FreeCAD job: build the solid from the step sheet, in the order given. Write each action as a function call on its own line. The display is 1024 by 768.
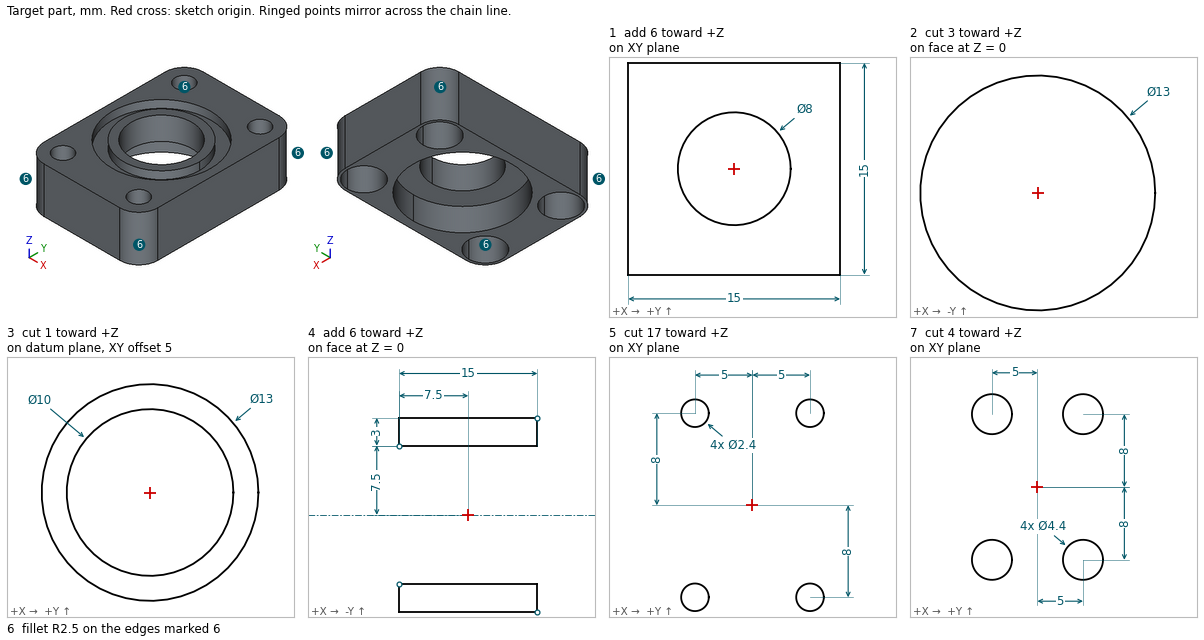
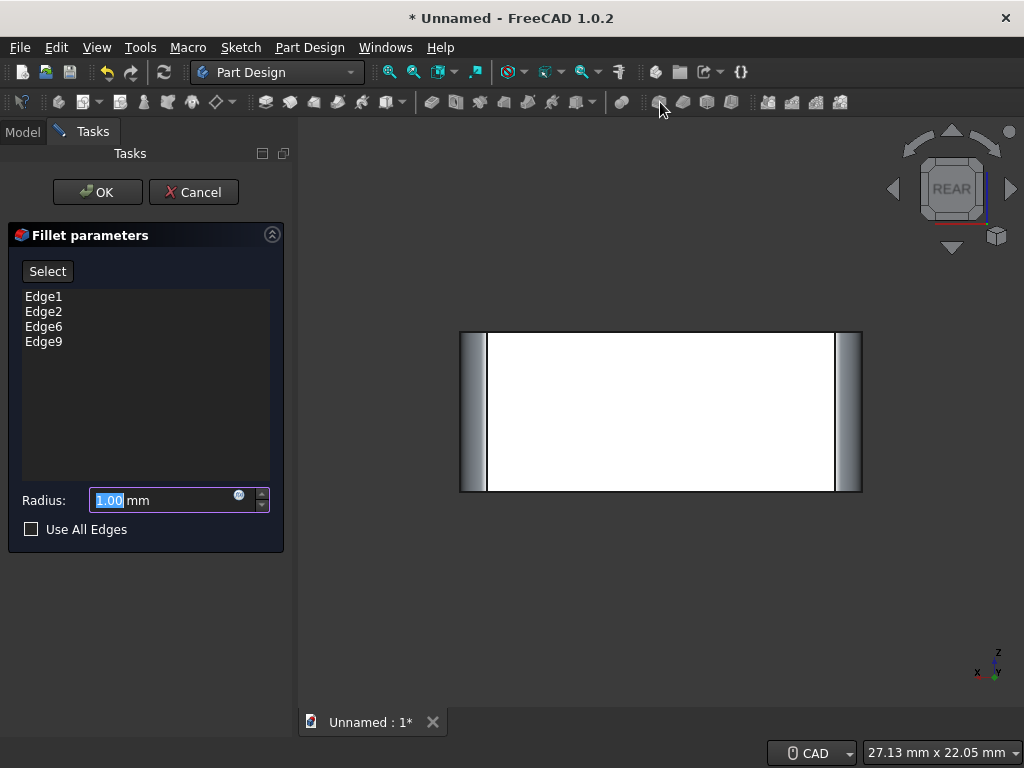
text(2.5)
key(Tab)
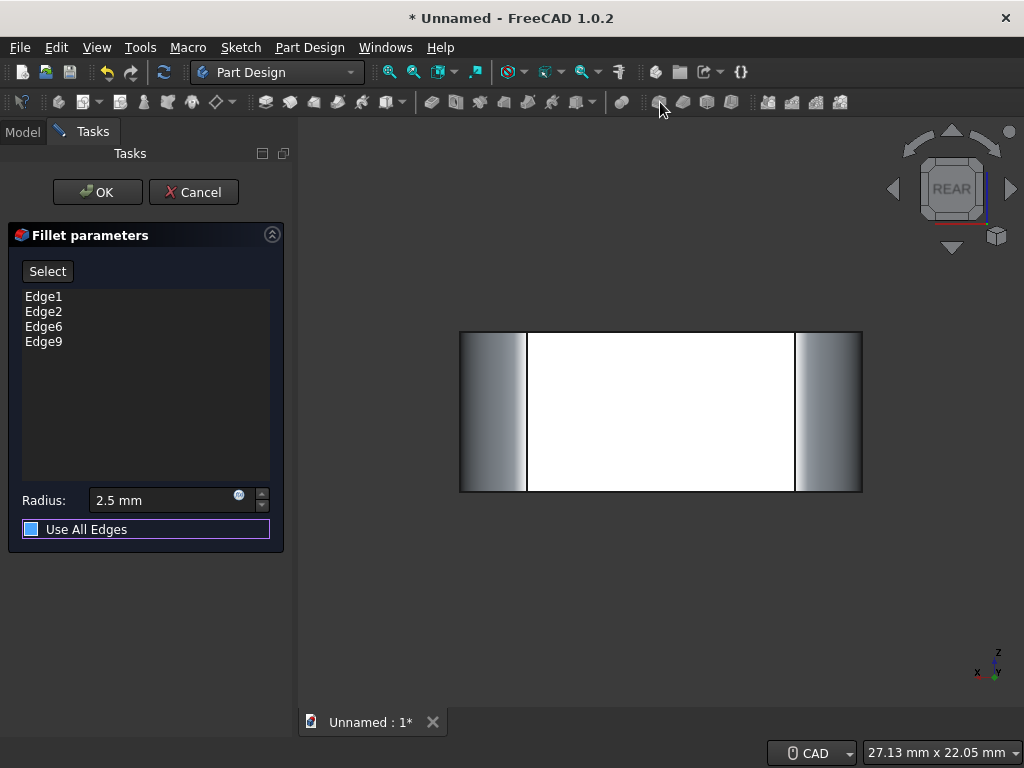
click(98, 192)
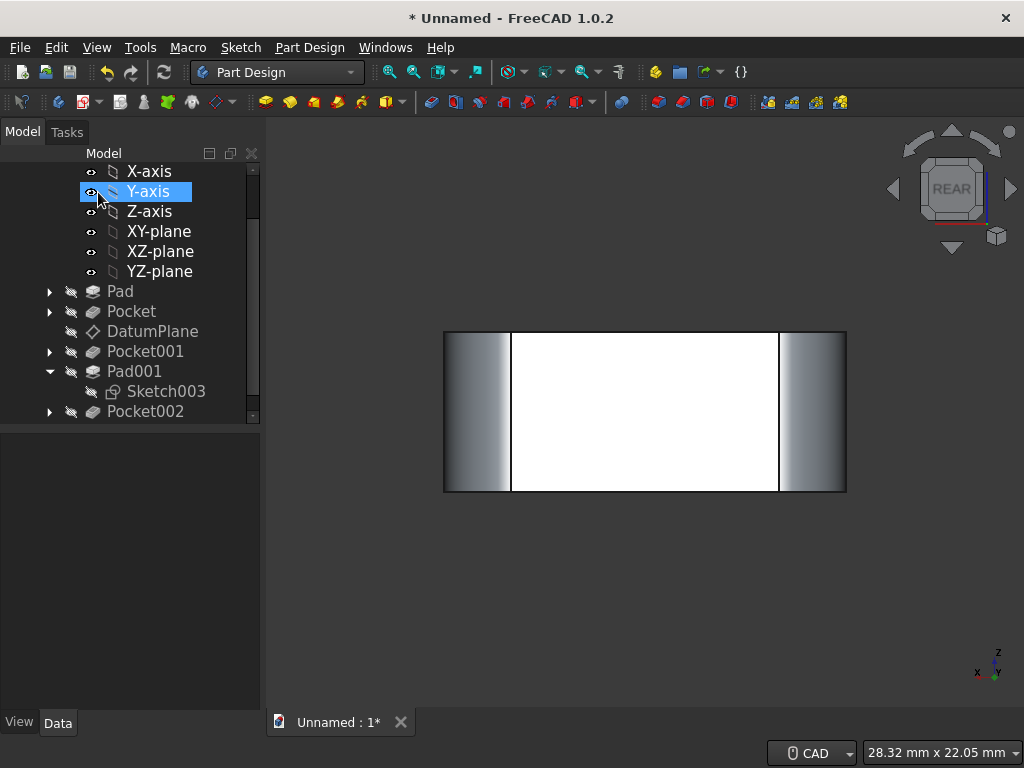
click(84, 102)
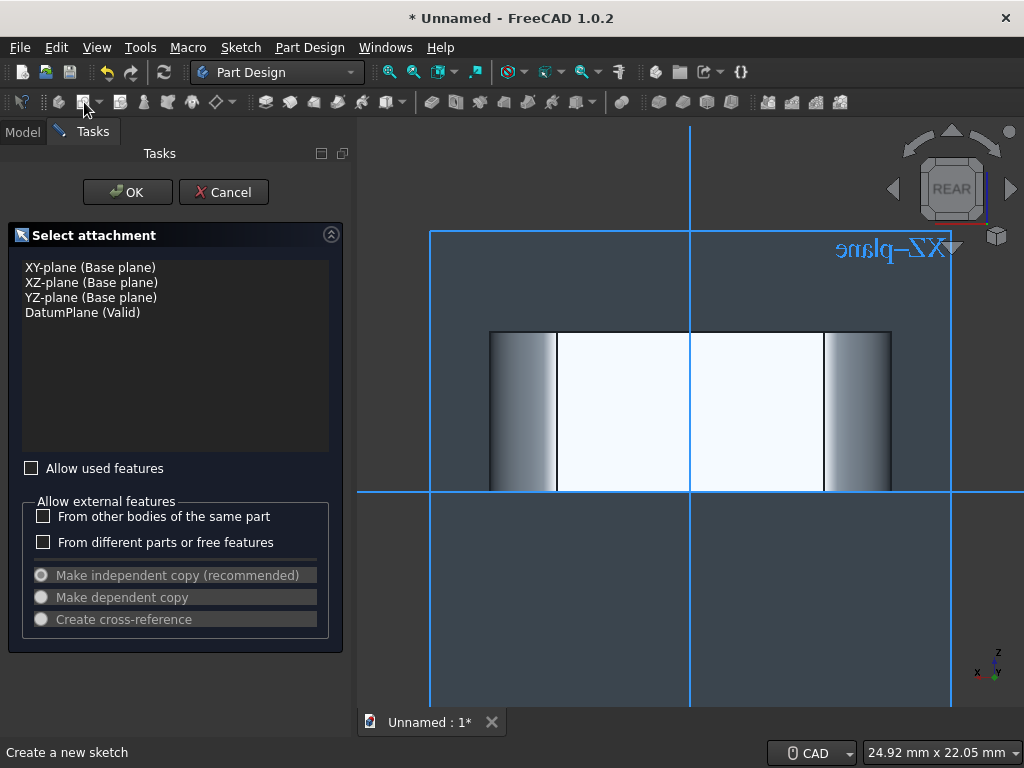
click(82, 268)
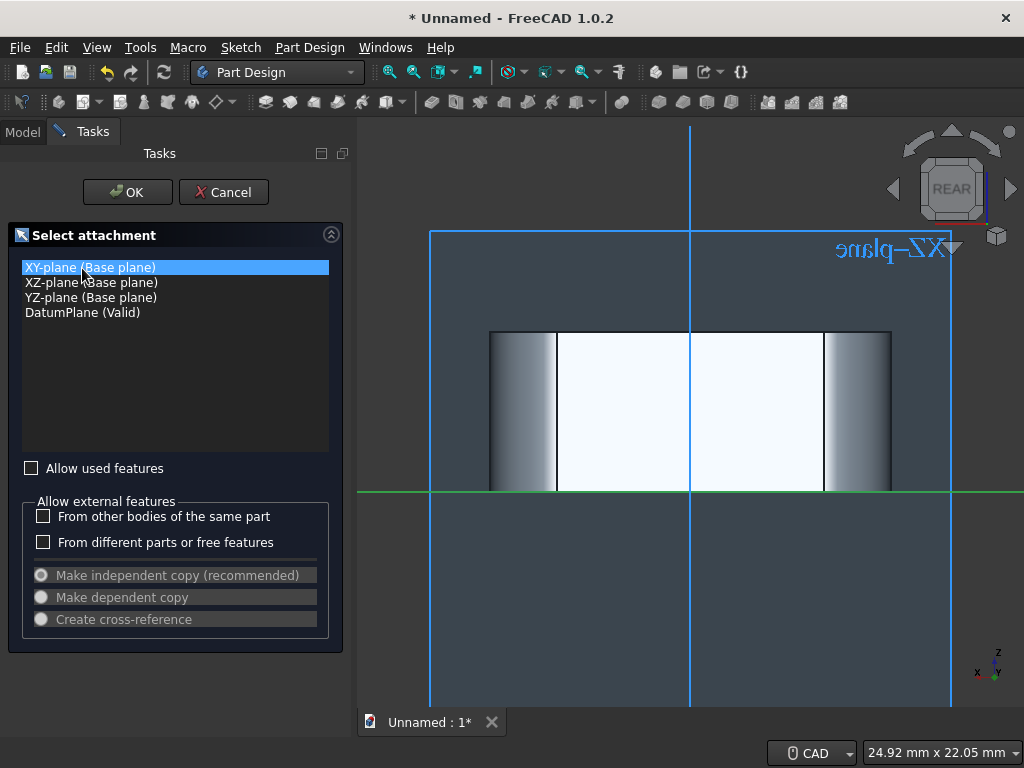
click(128, 192)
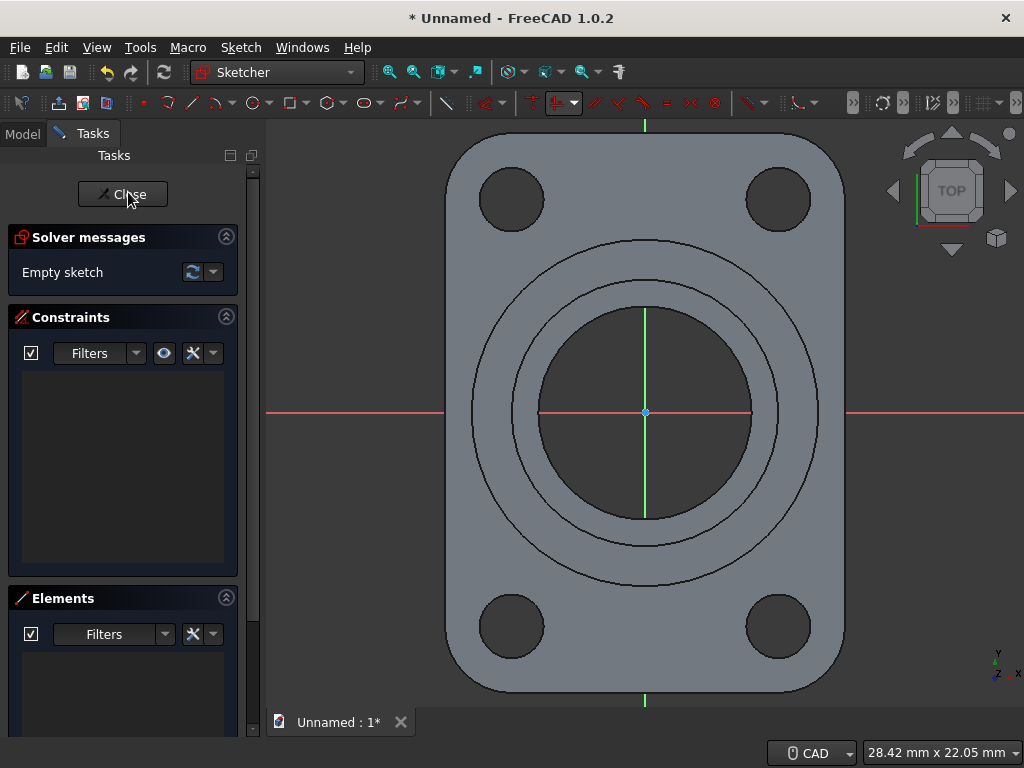
click(108, 104)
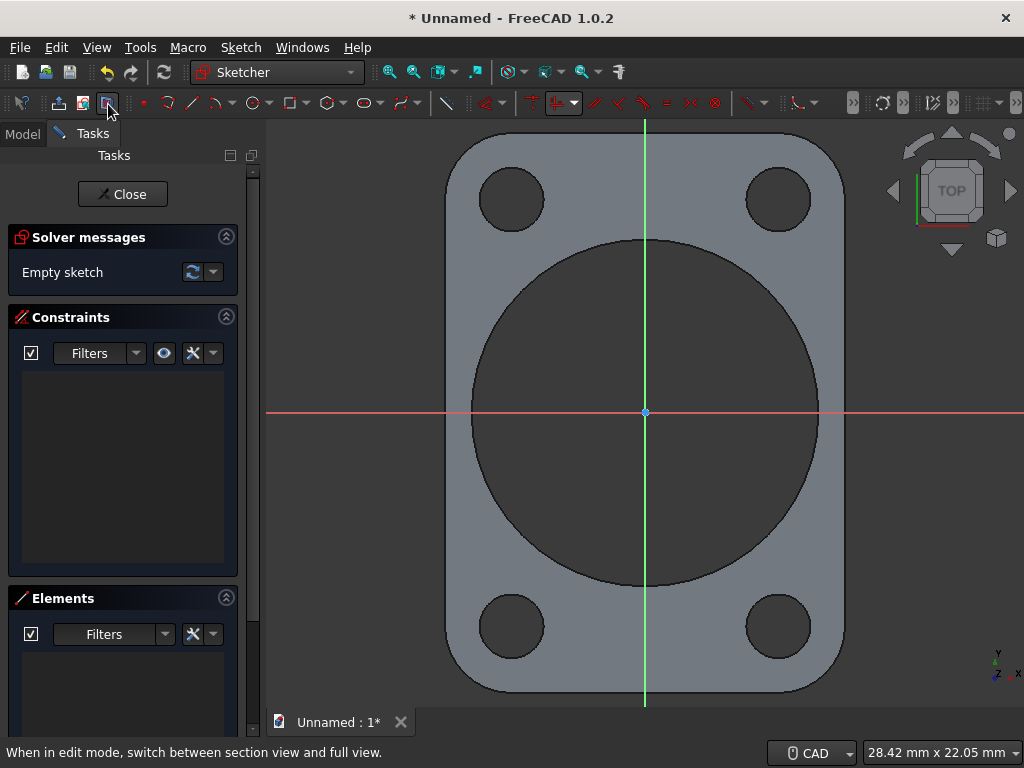
scroll(437, 413, down, 2)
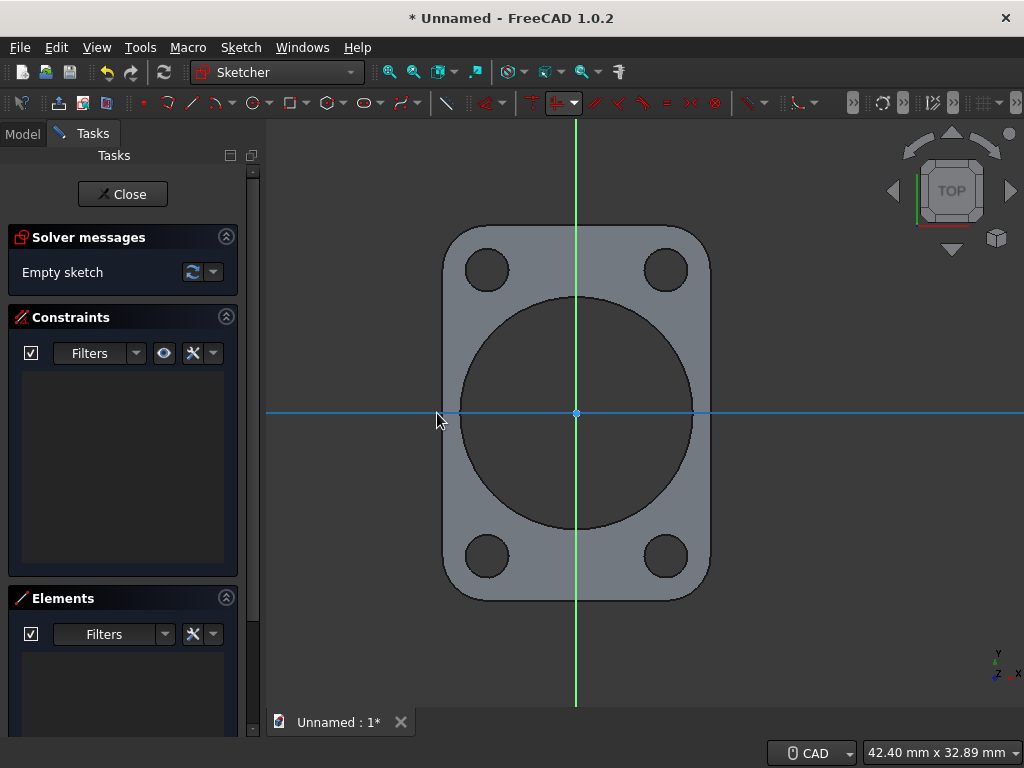
click(254, 104)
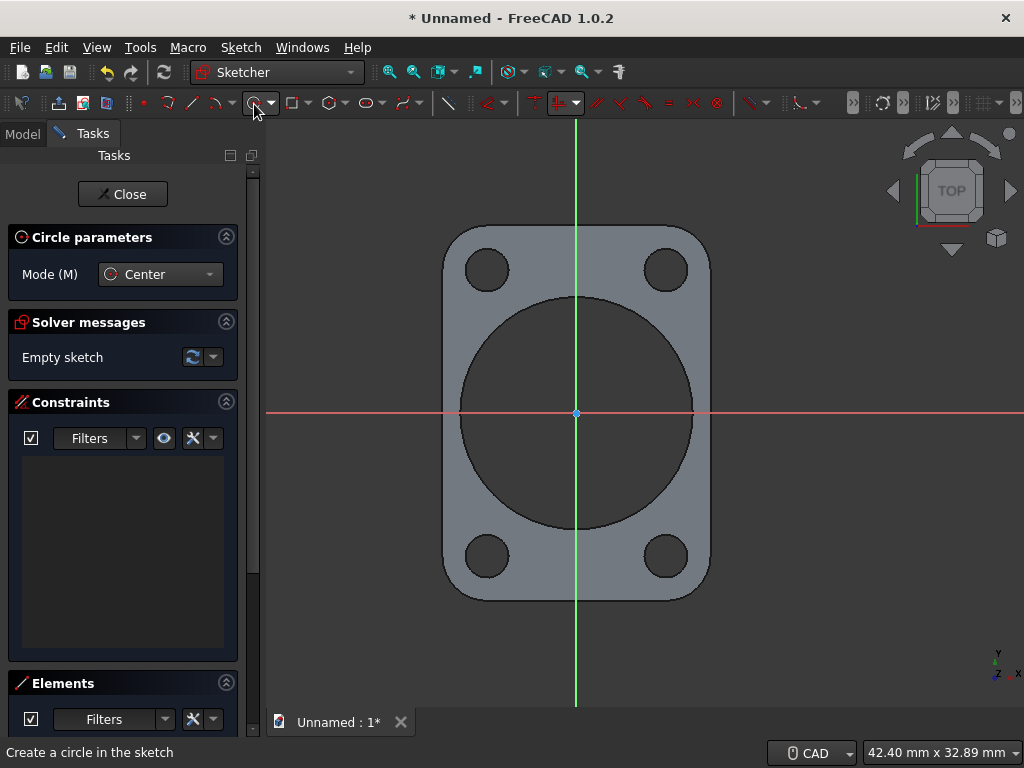
click(666, 556)
click(694, 528)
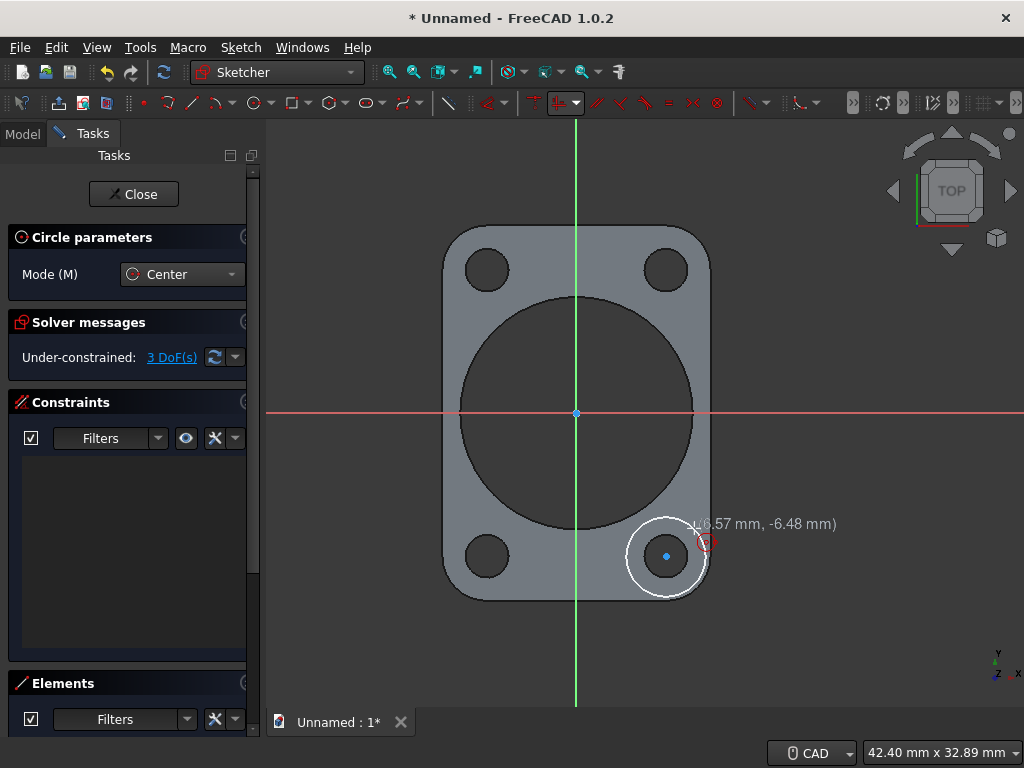
click(666, 270)
click(694, 242)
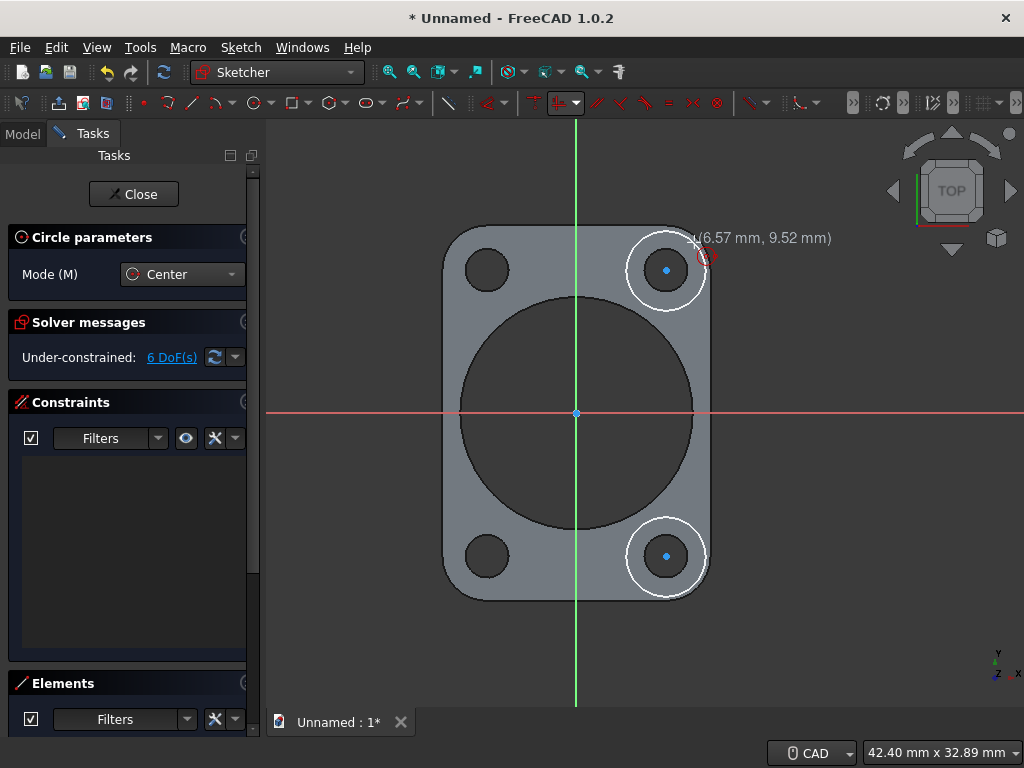
click(487, 270)
click(515, 242)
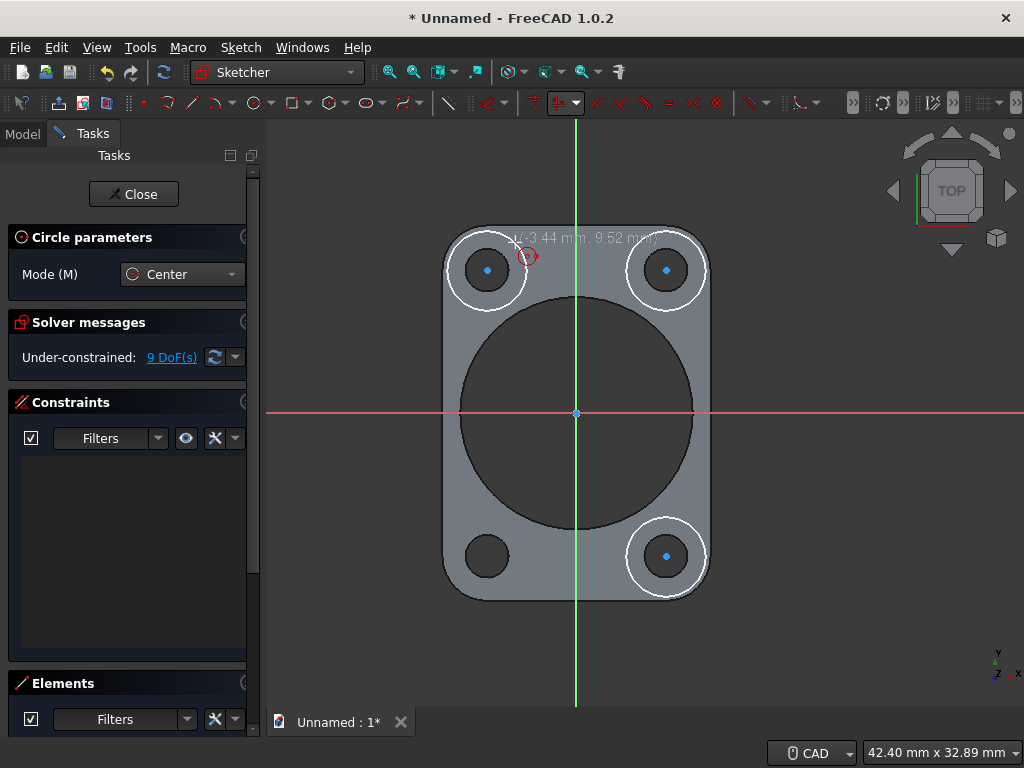
click(487, 556)
click(515, 528)
key(Escape)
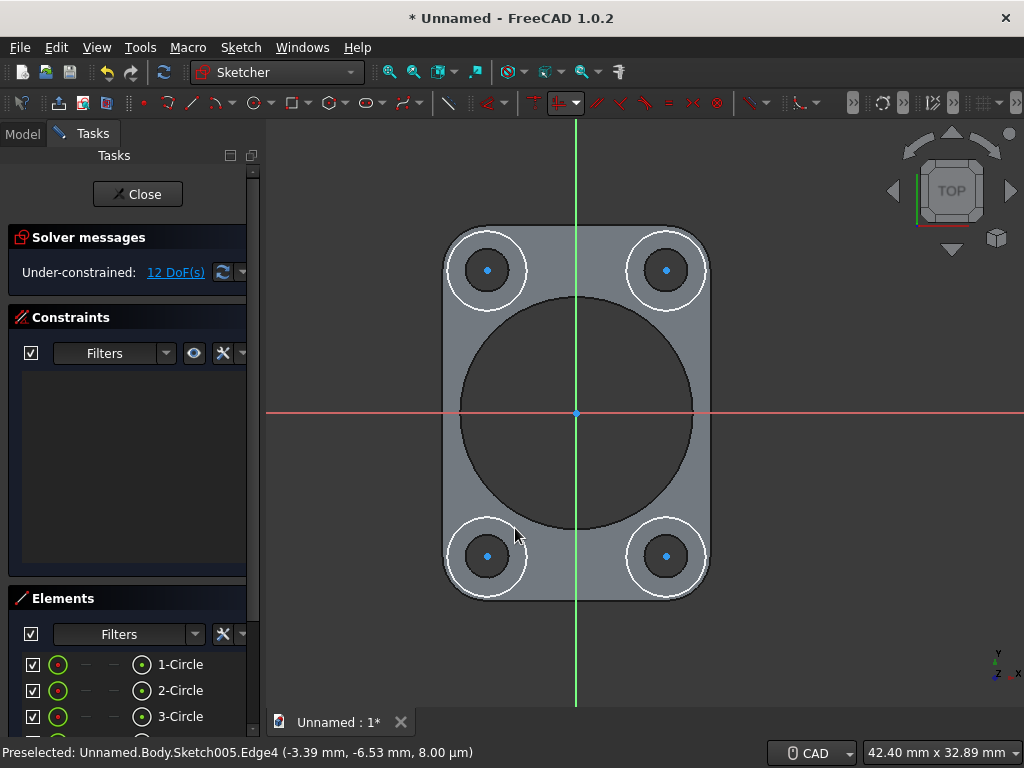
click(694, 529)